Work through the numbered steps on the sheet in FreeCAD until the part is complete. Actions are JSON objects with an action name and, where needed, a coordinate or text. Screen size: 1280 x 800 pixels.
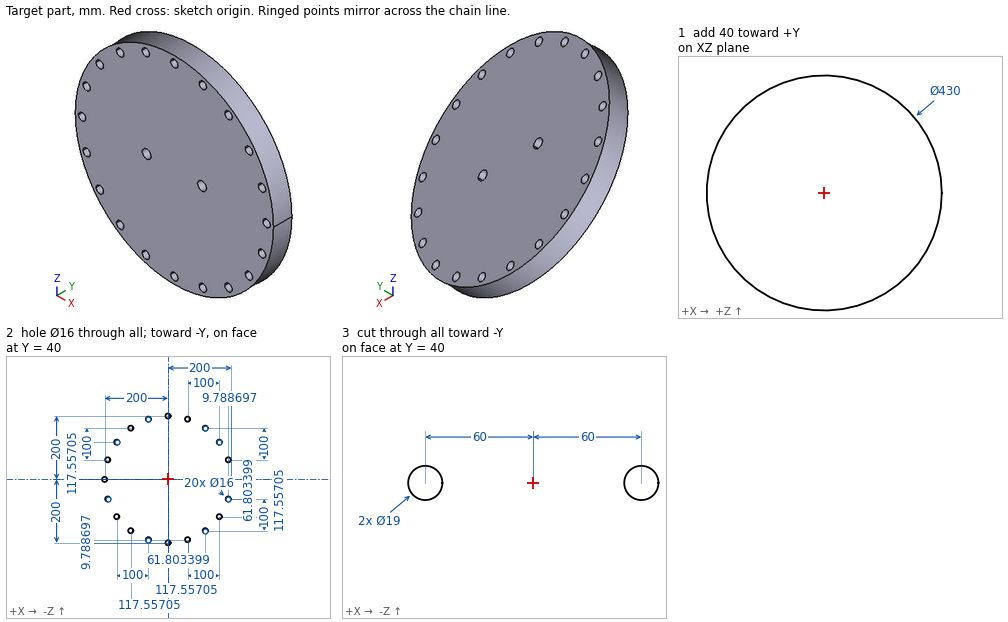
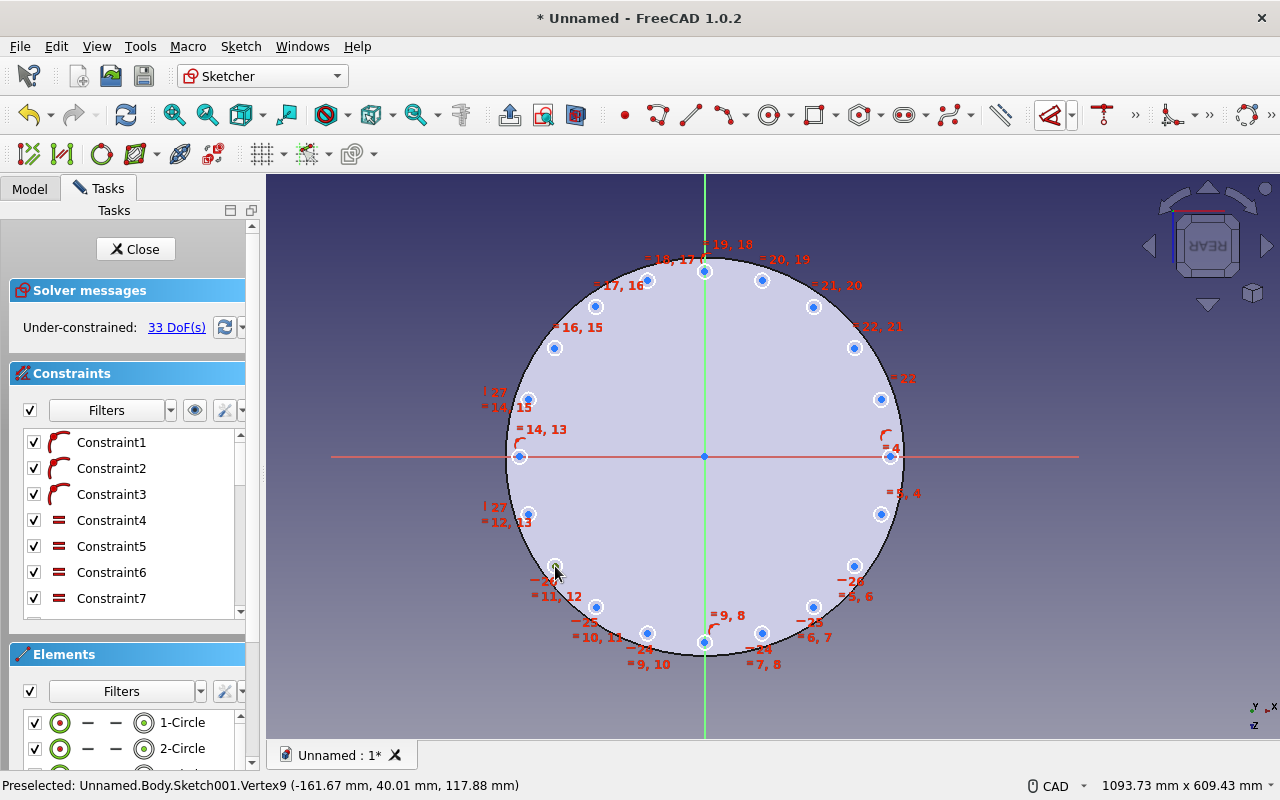
{"action": "left_click", "coordinate": [555, 348]}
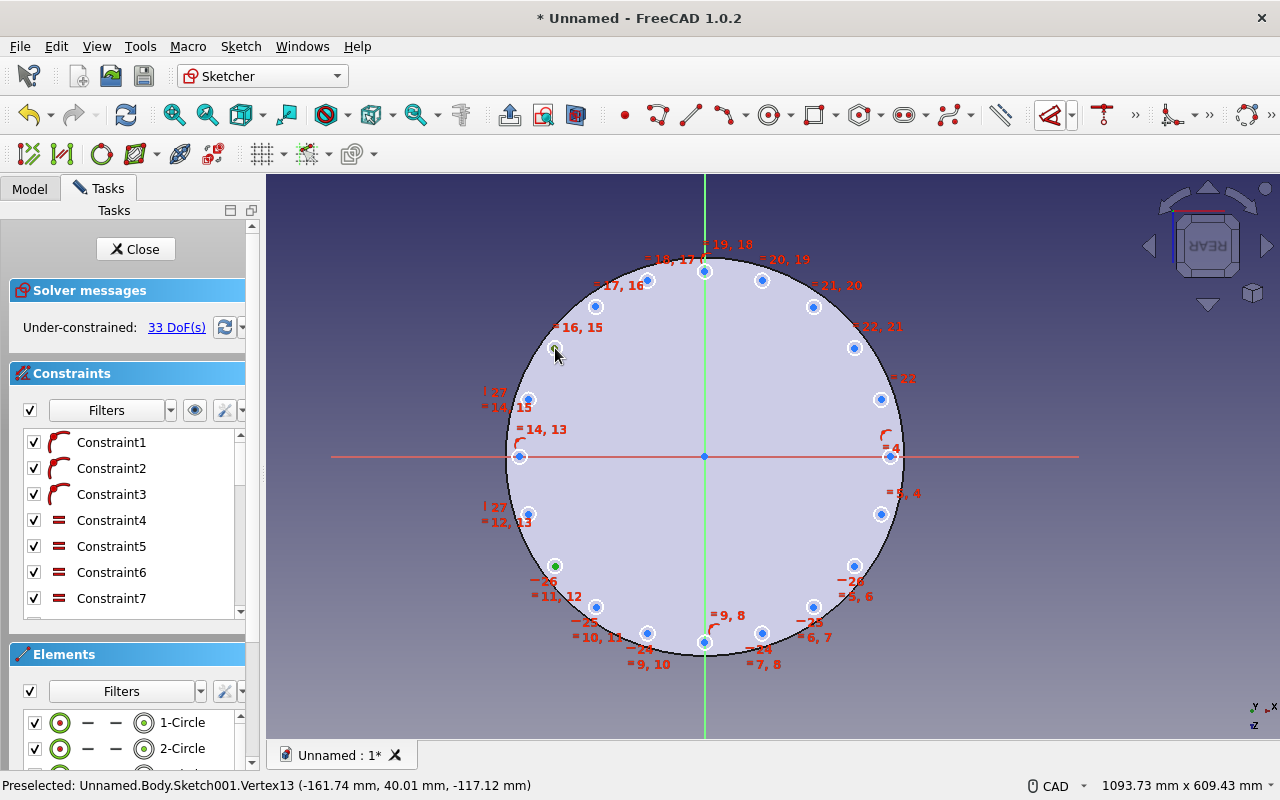
{"action": "key", "text": "v"}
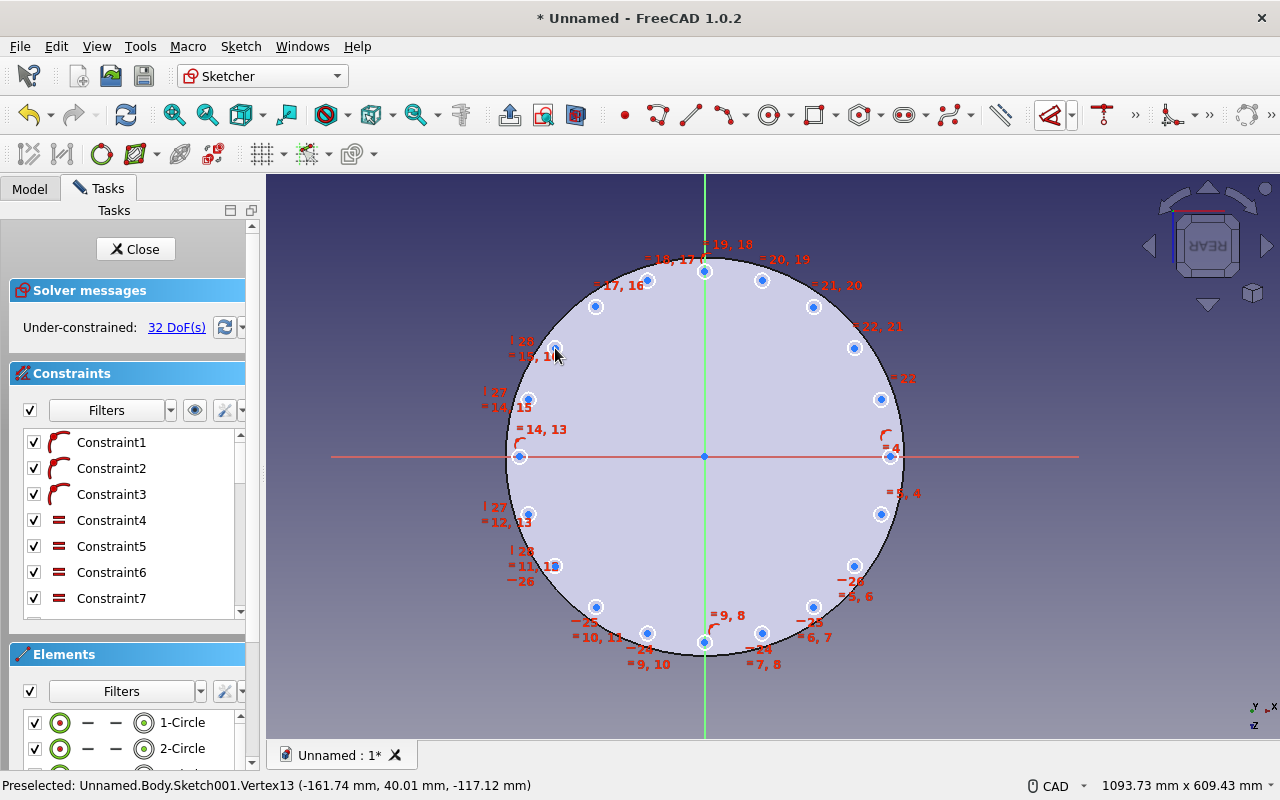
{"action": "left_click", "coordinate": [596, 607]}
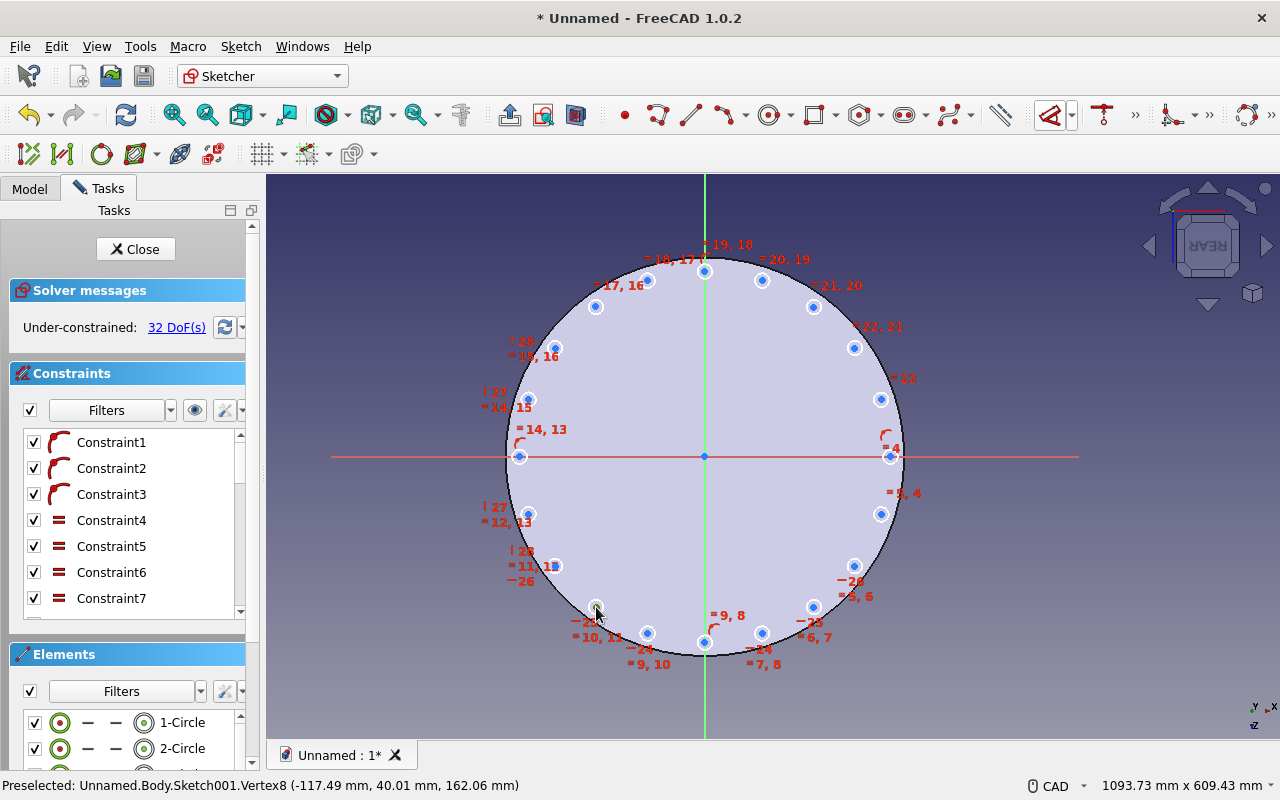
{"action": "left_click", "coordinate": [596, 307]}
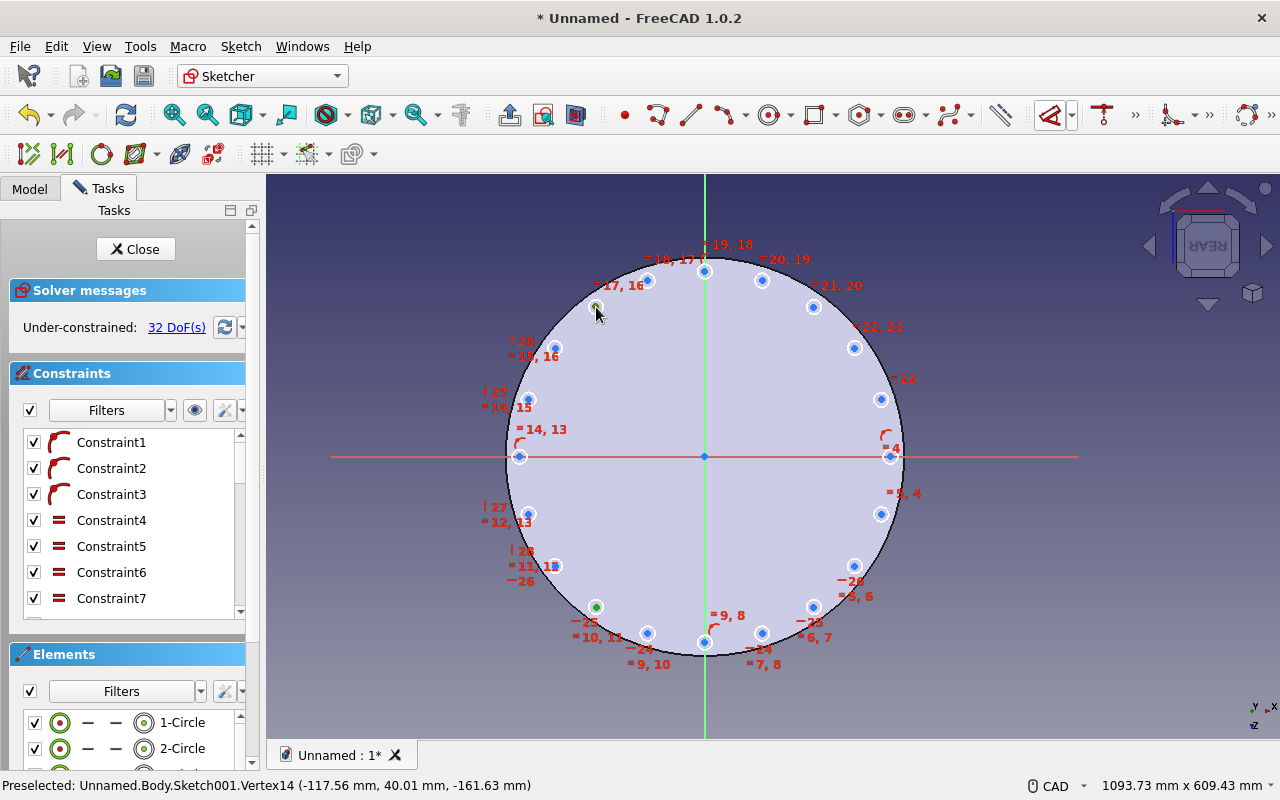
{"action": "key", "text": "v"}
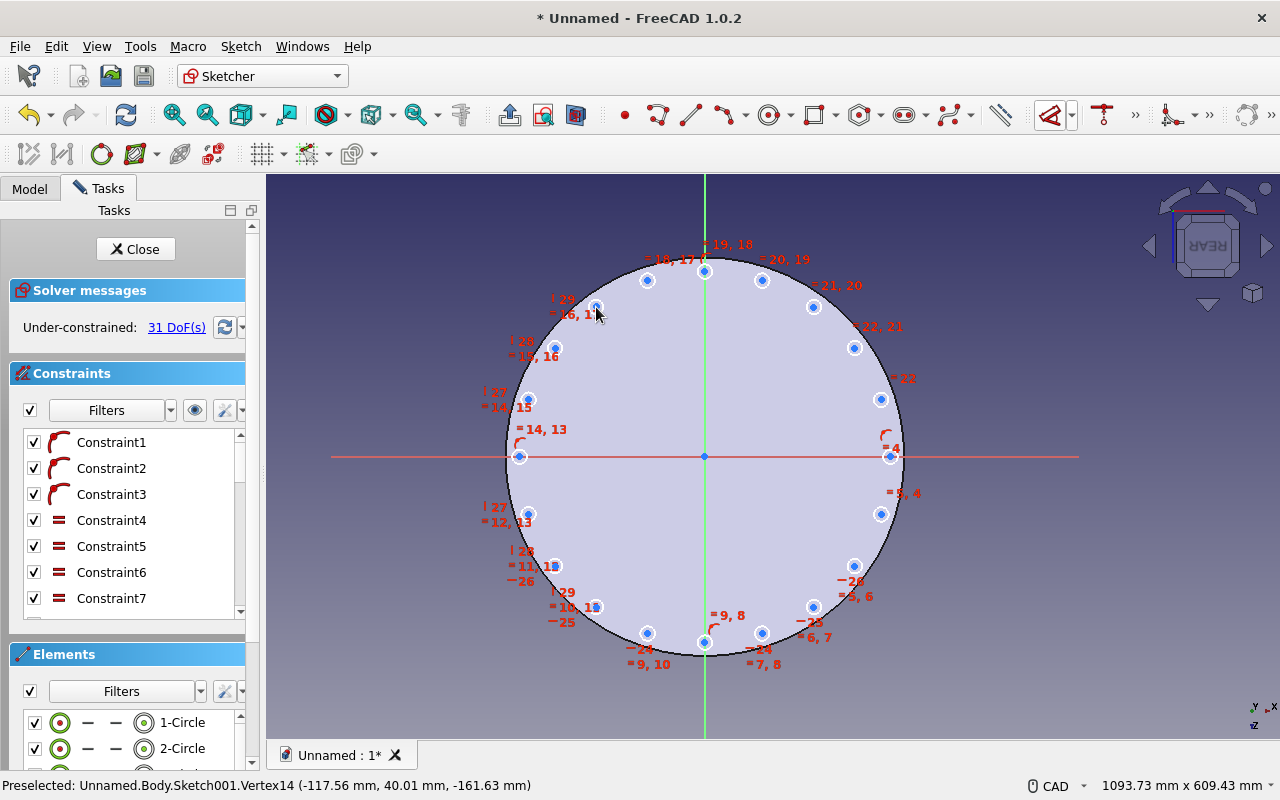
{"action": "left_click", "coordinate": [648, 281]}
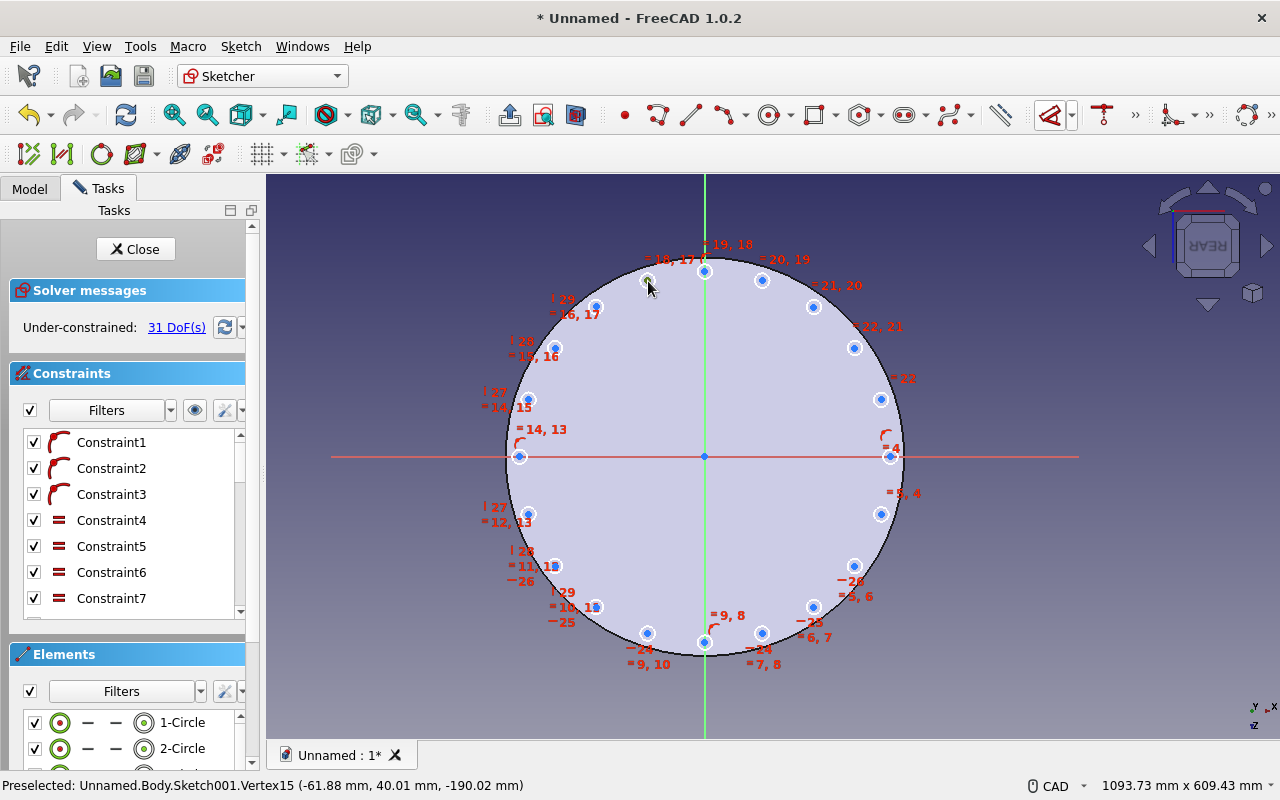
{"action": "left_click", "coordinate": [762, 281]}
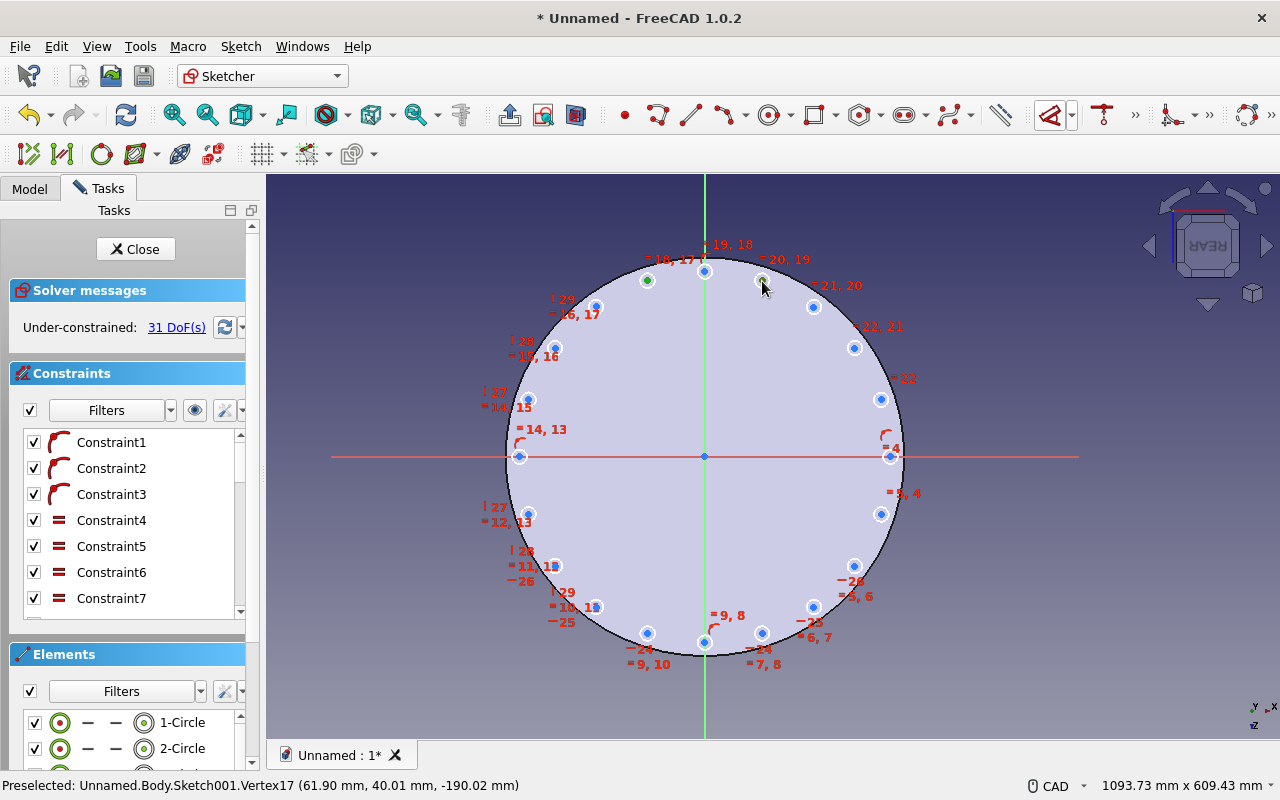
{"action": "key", "text": "h"}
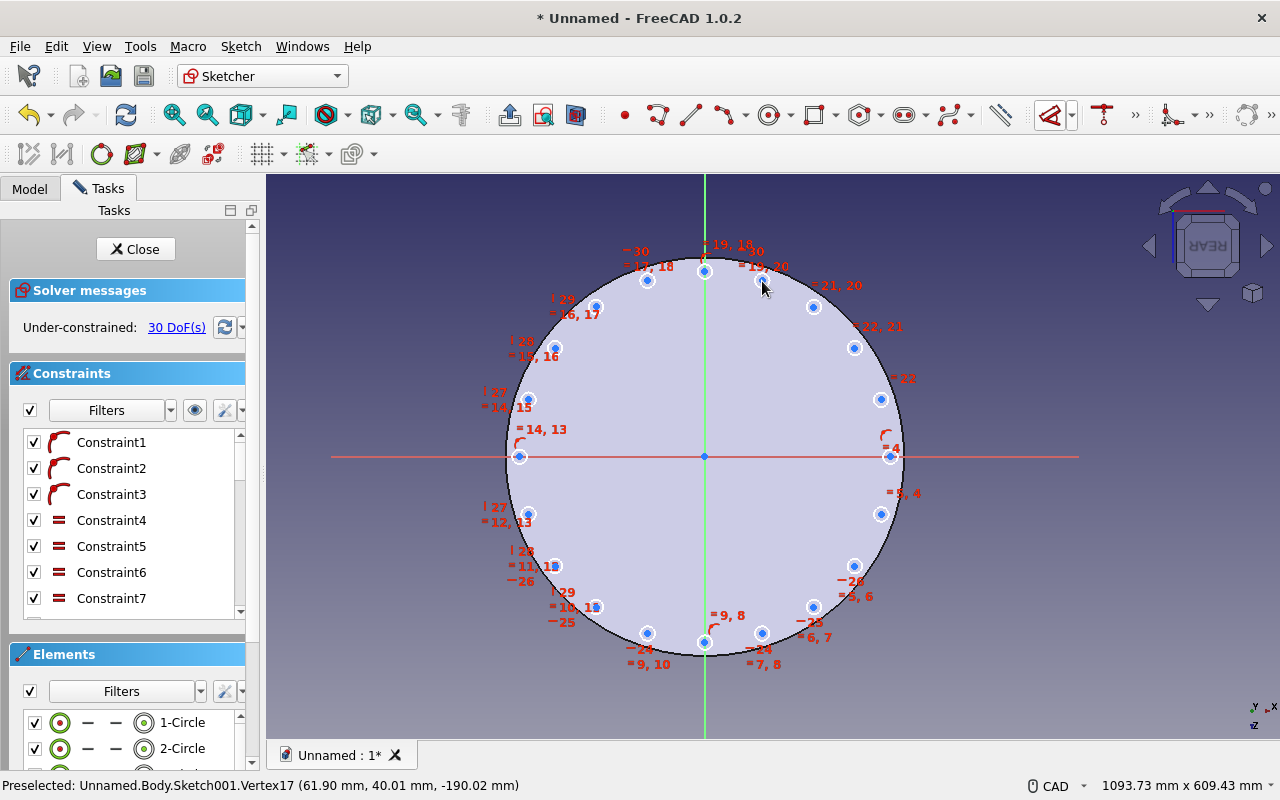
{"action": "scroll", "coordinate": [596, 307], "scroll_direction": "up", "scroll_amount": 4}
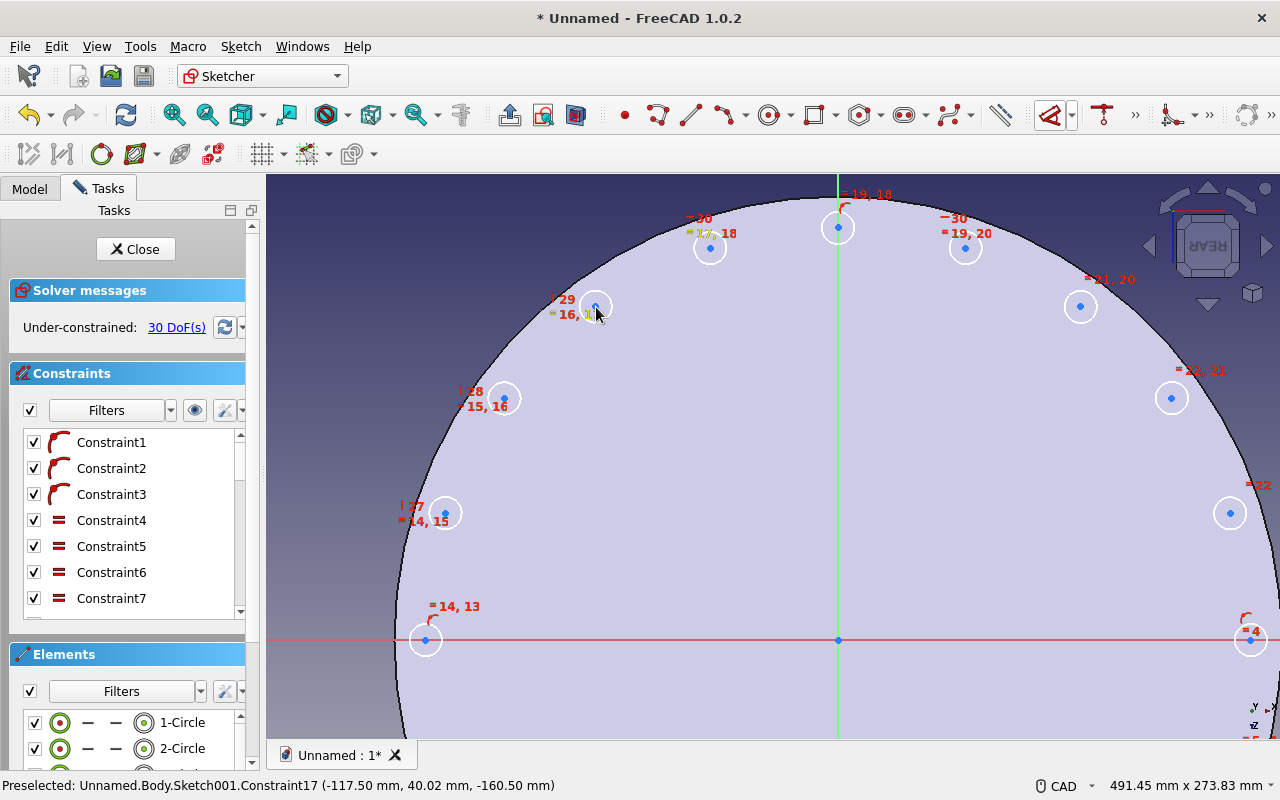
{"action": "scroll", "coordinate": [596, 307], "scroll_direction": "up", "scroll_amount": 4}